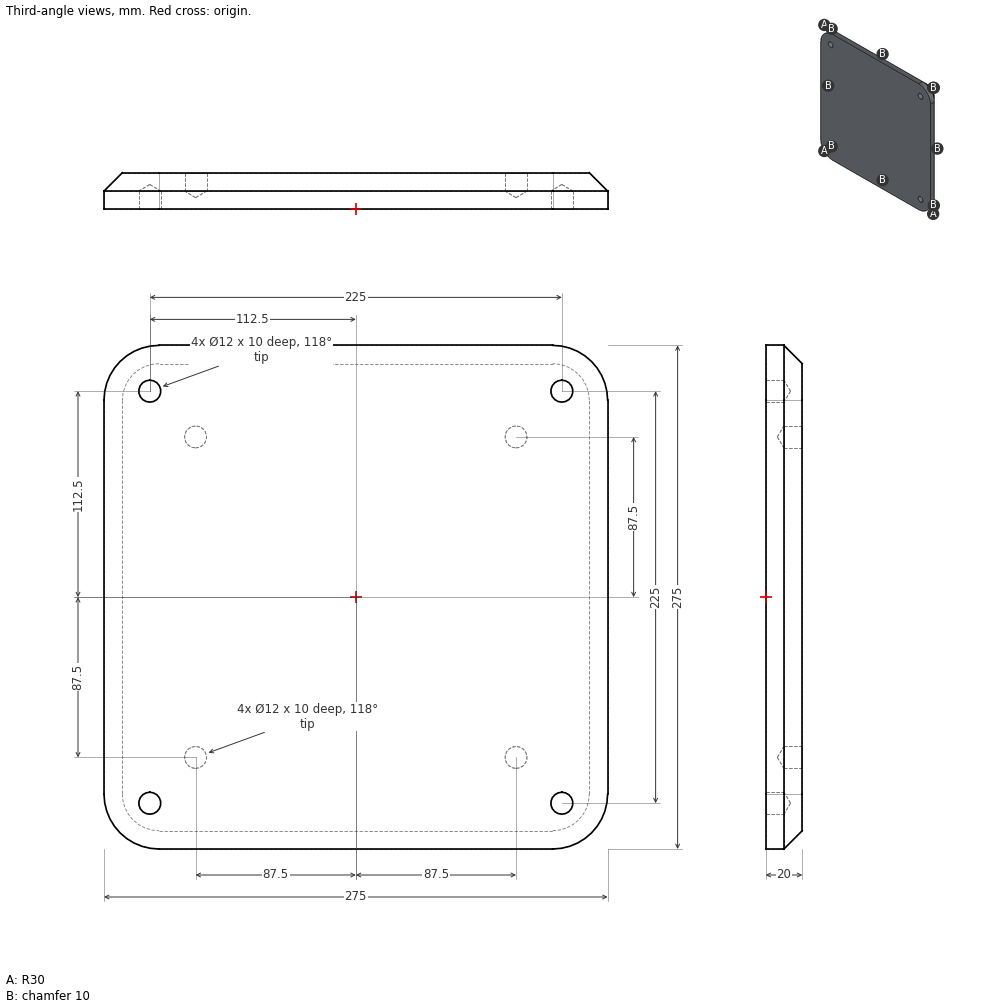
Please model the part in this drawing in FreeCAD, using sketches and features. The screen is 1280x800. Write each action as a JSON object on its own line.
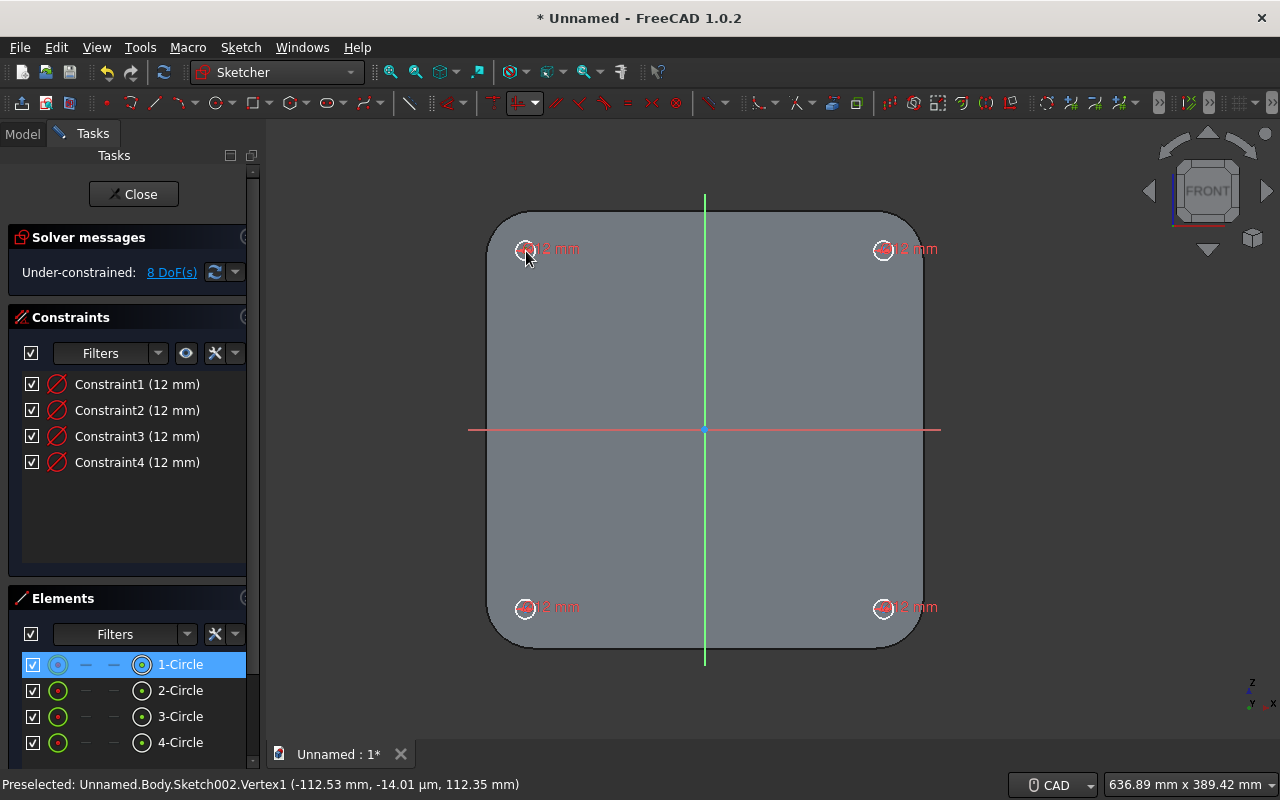
{"action": "left_click", "coordinate": [884, 251]}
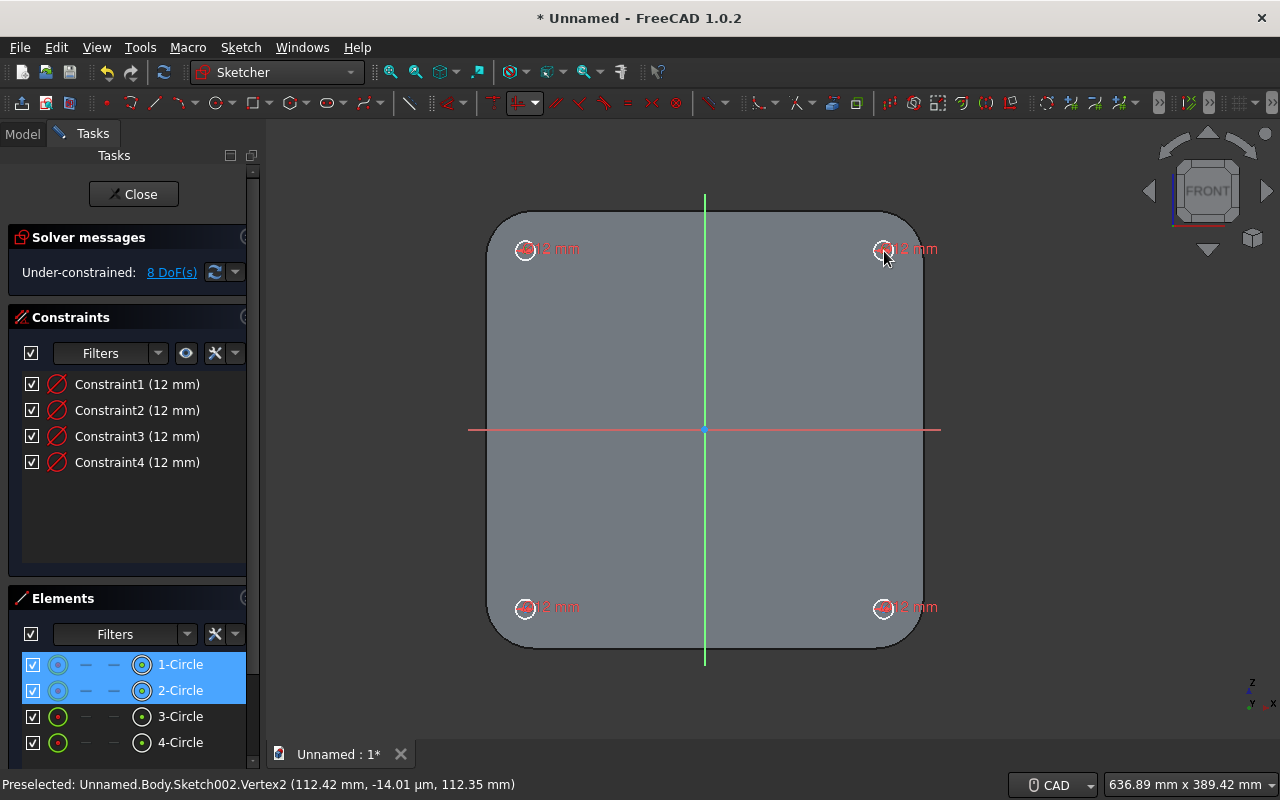
{"action": "key", "text": "h"}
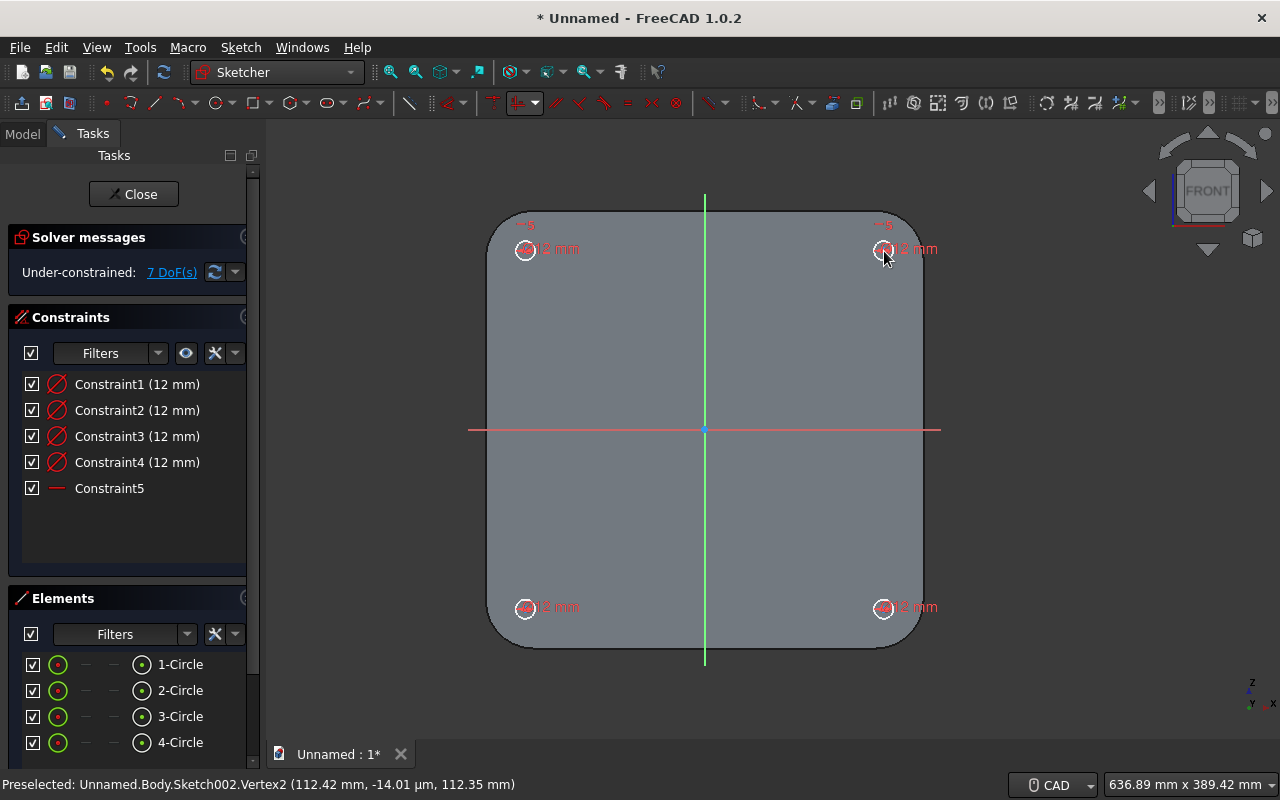
{"action": "left_click", "coordinate": [884, 251]}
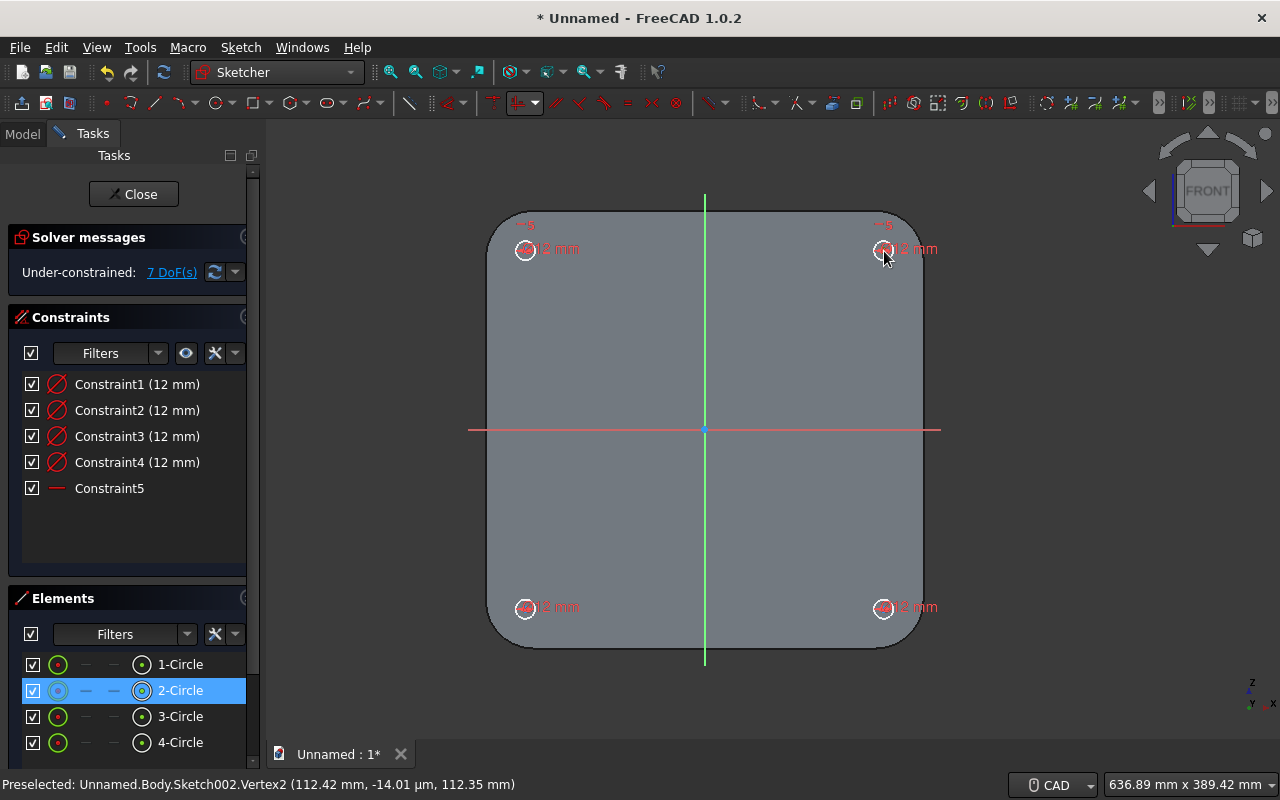
{"action": "left_click", "coordinate": [884, 609]}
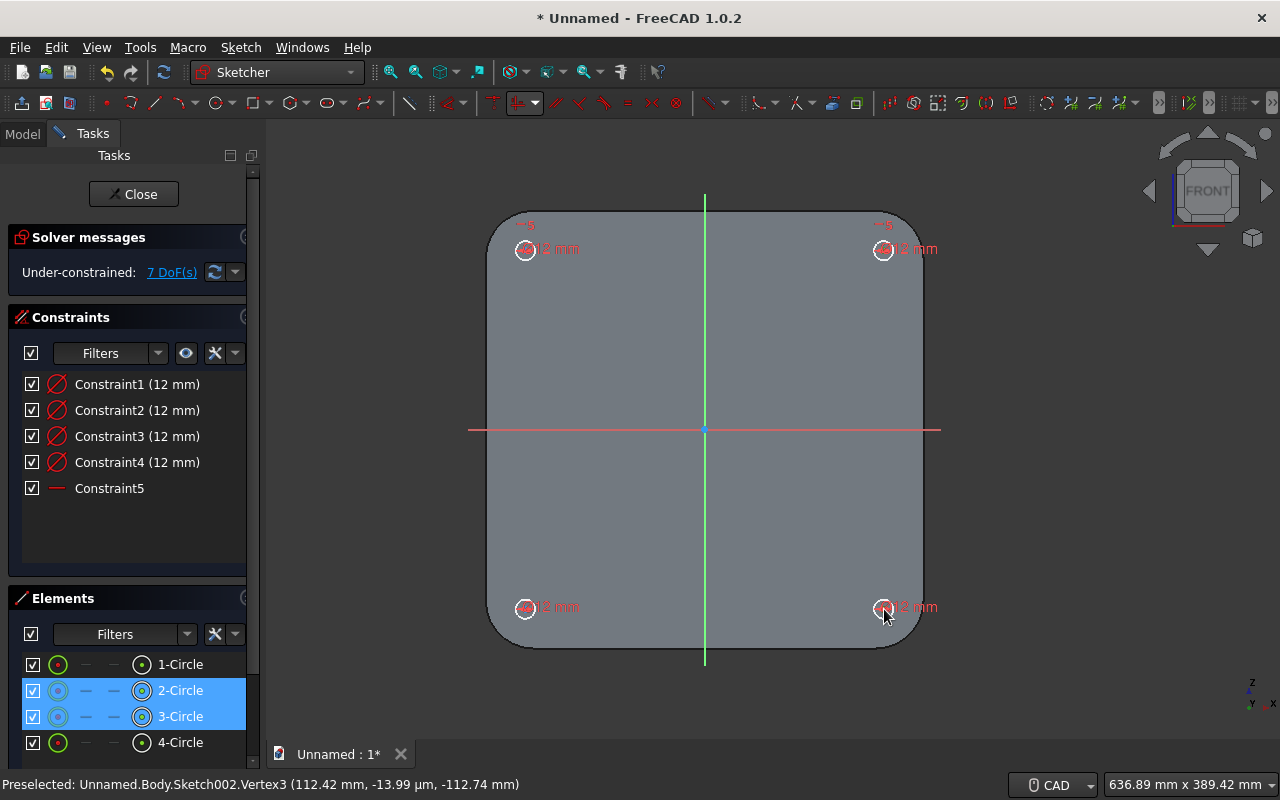
{"action": "key", "text": "v"}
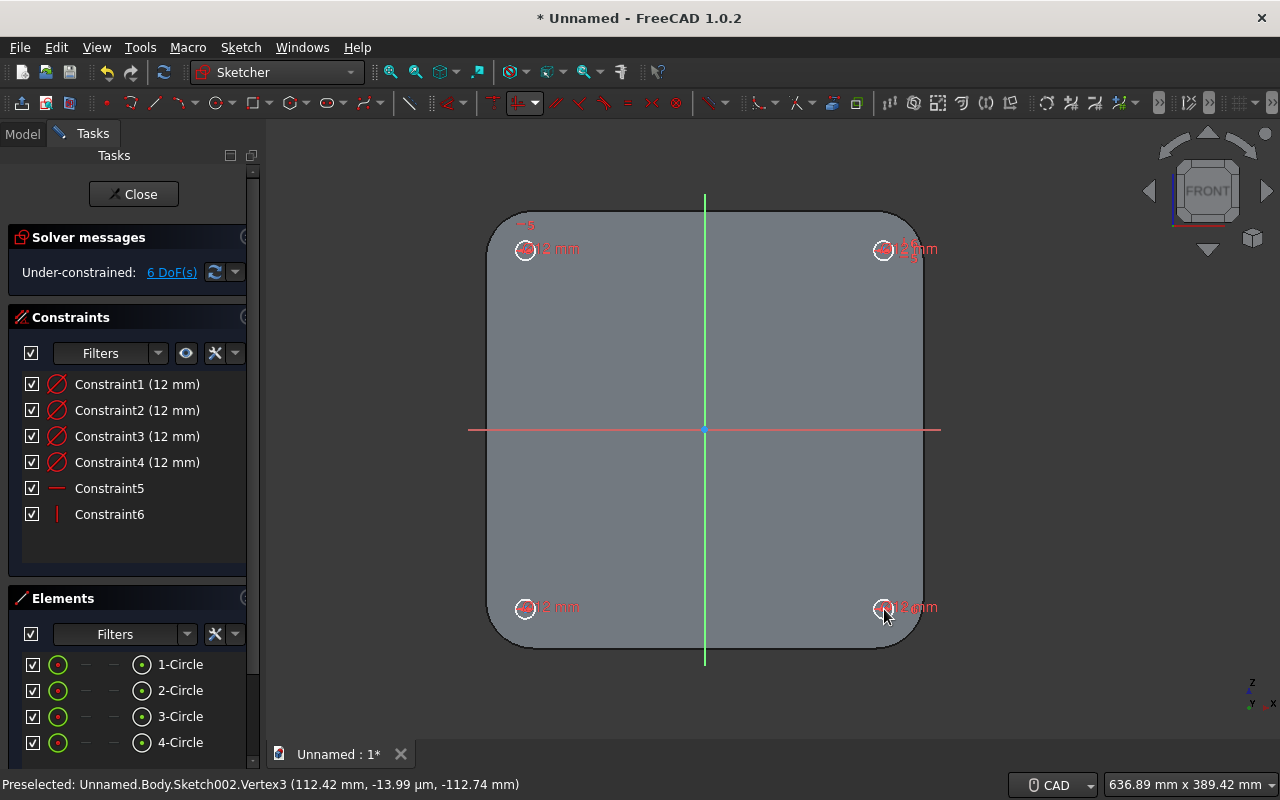
{"action": "left_click", "coordinate": [526, 251]}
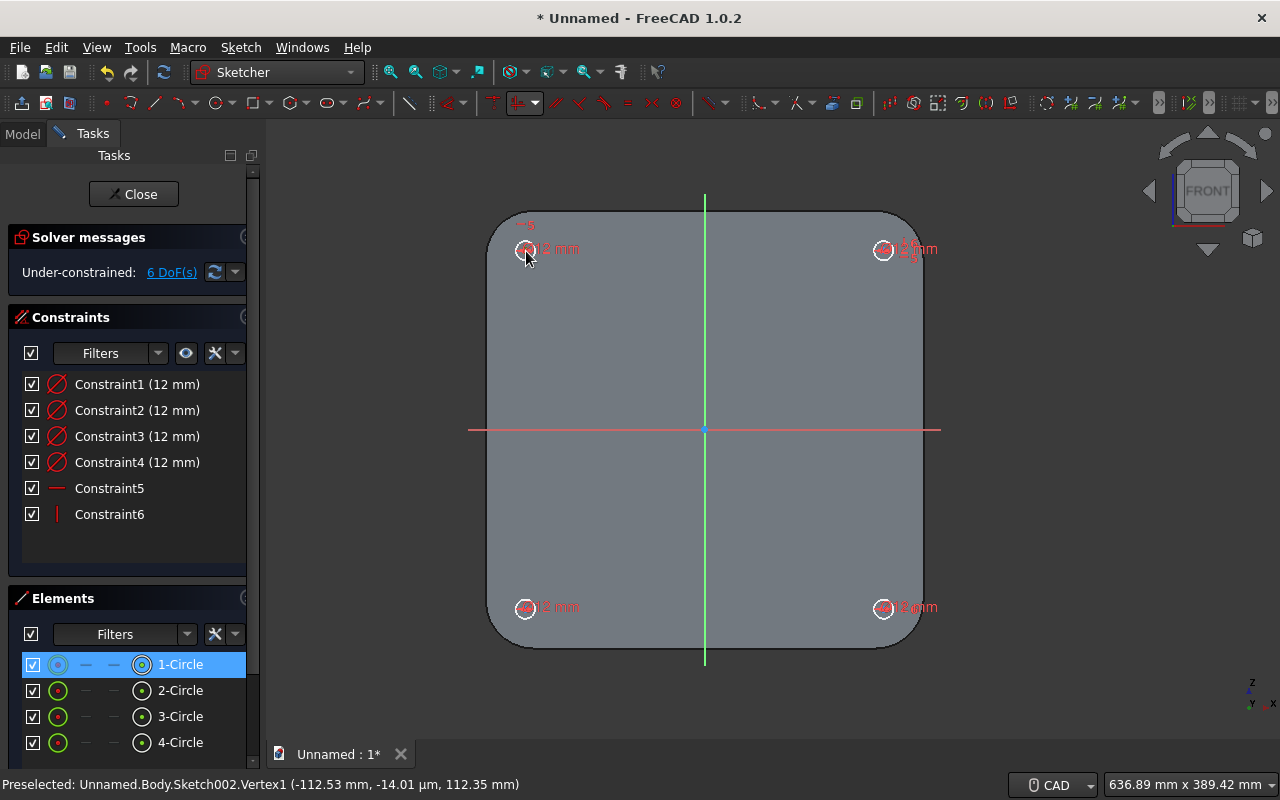
{"action": "left_click", "coordinate": [525, 609]}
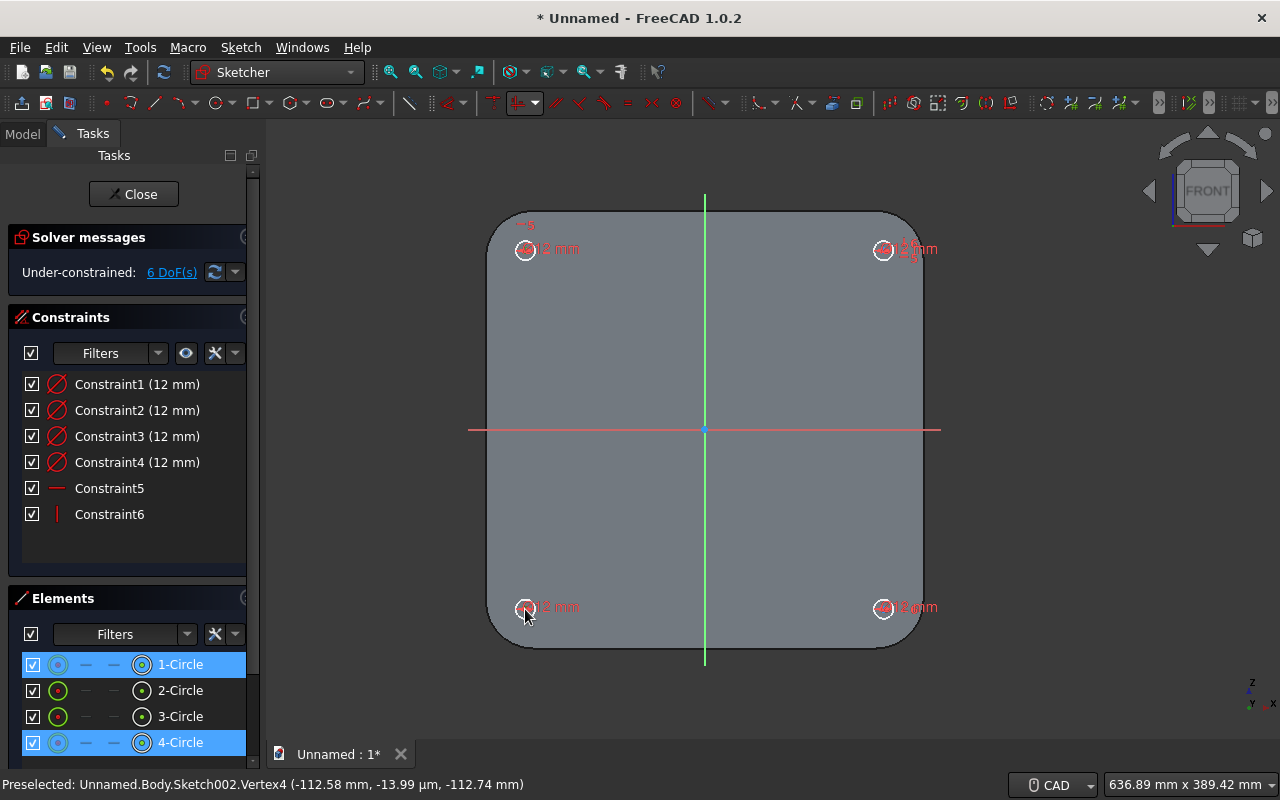
{"action": "left_click", "coordinate": [538, 104]}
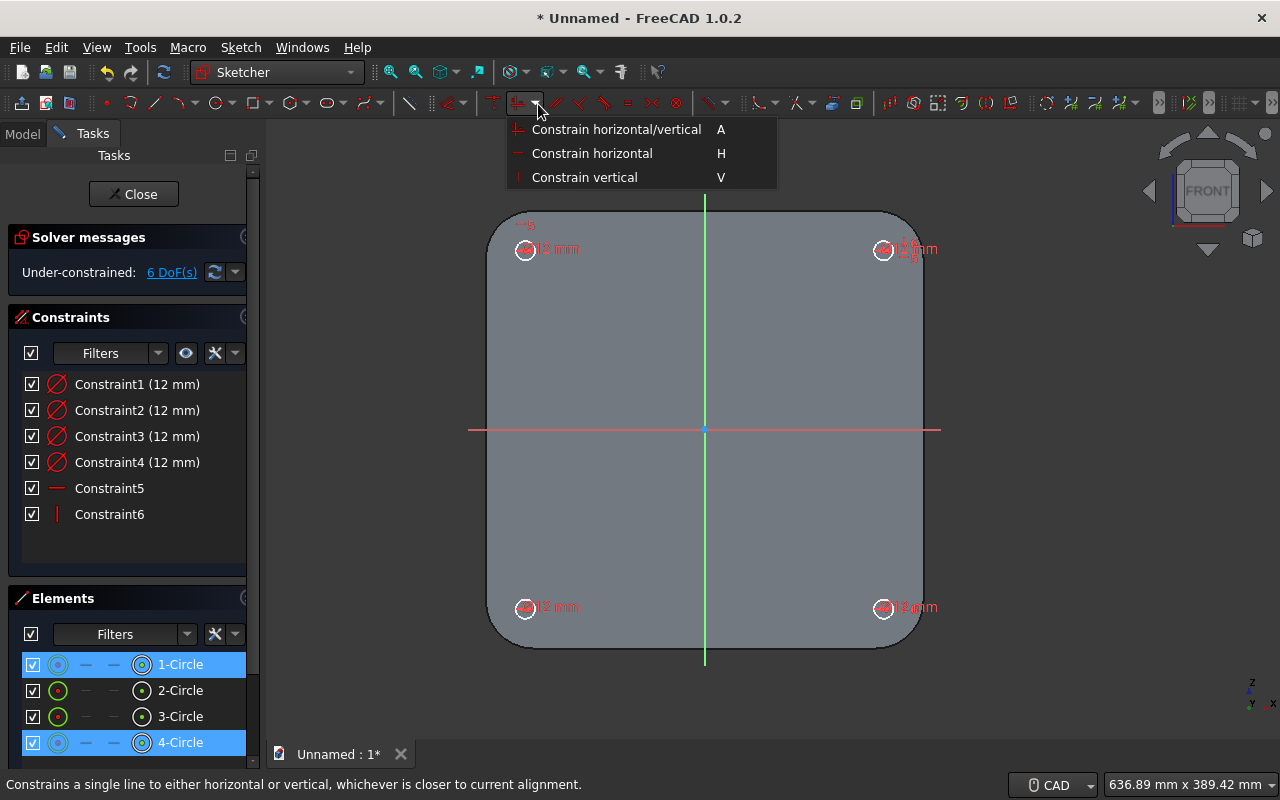
{"action": "left_click", "coordinate": [642, 177]}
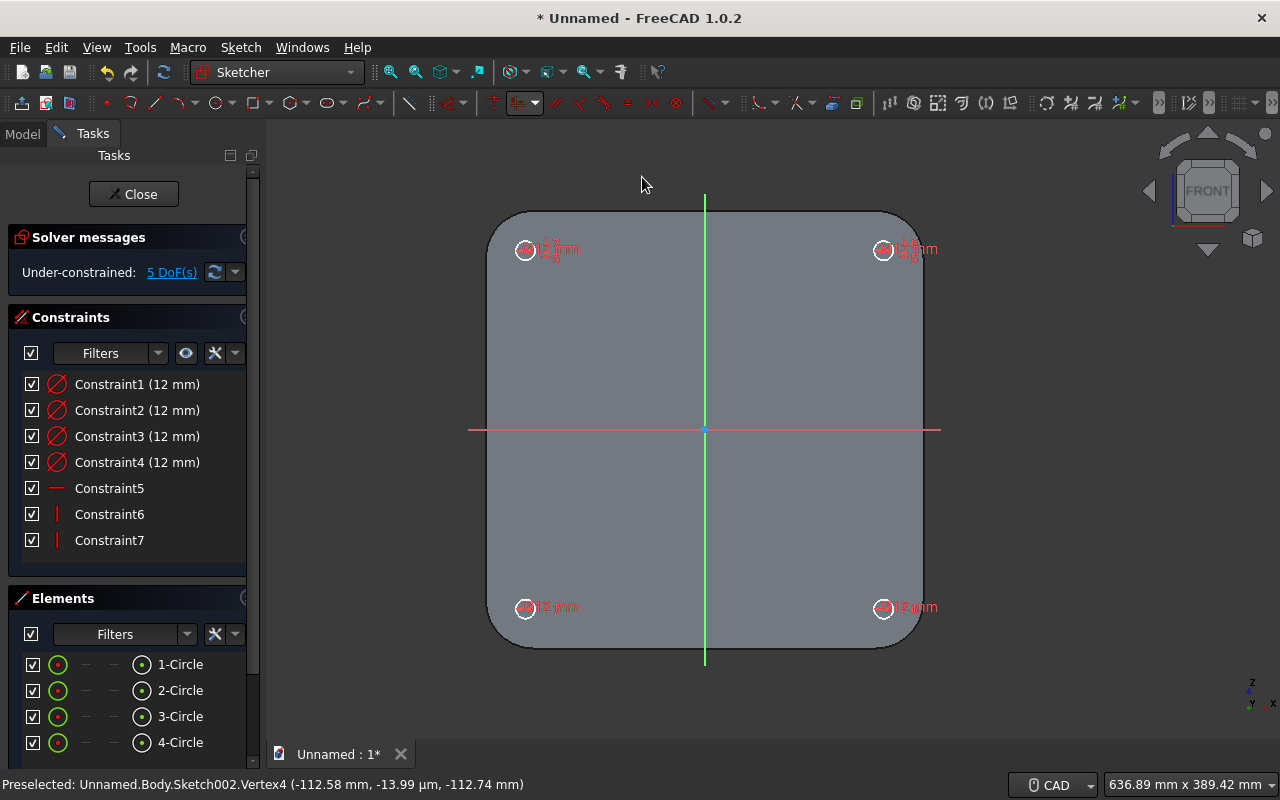
{"action": "left_click", "coordinate": [884, 609]}